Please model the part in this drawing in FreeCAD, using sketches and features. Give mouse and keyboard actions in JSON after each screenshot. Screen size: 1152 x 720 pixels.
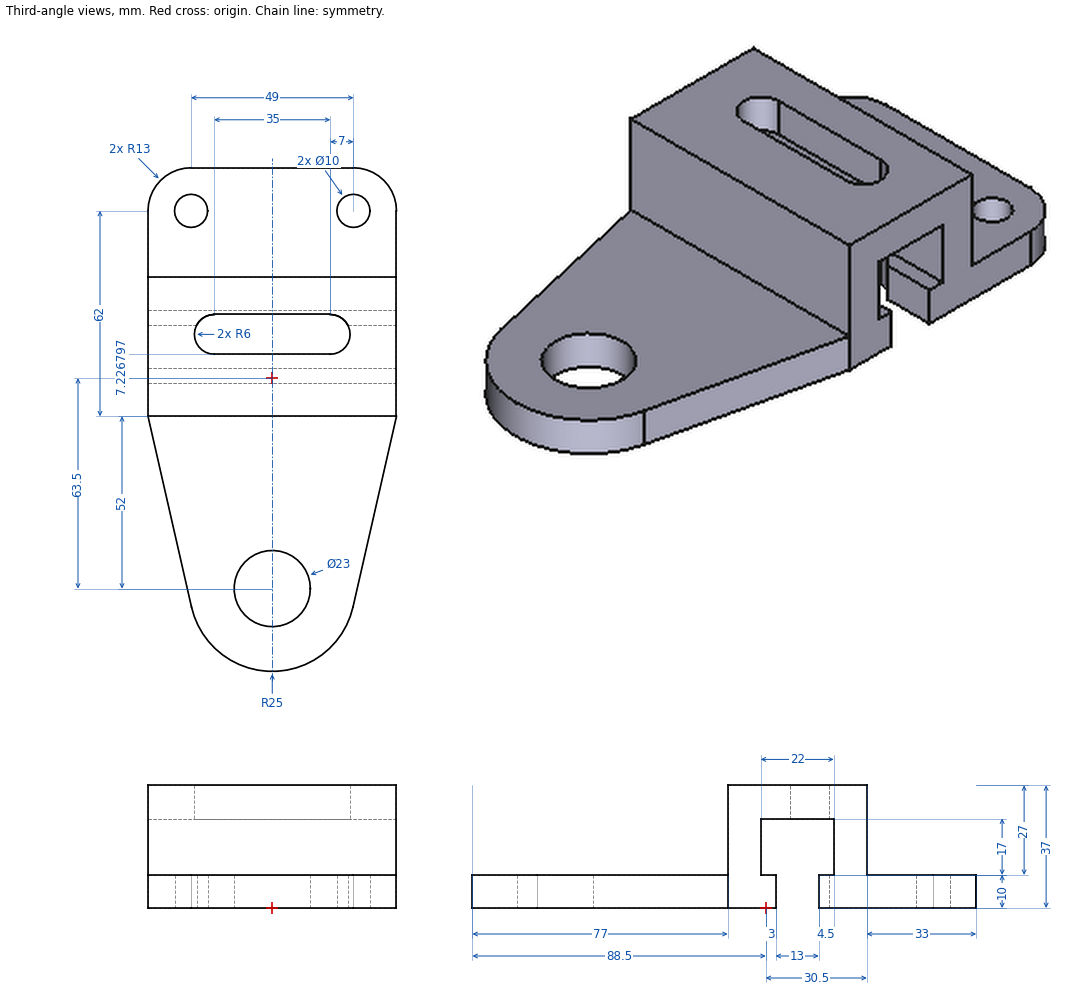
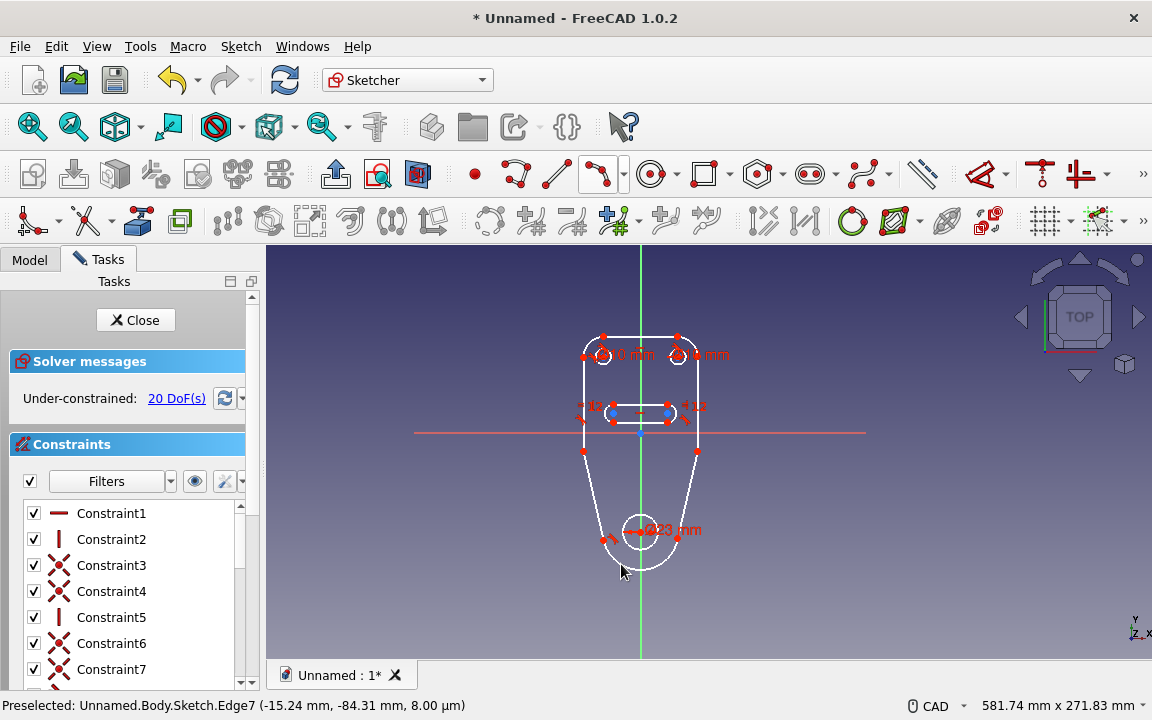
{"action": "left_click", "coordinate": [684, 513]}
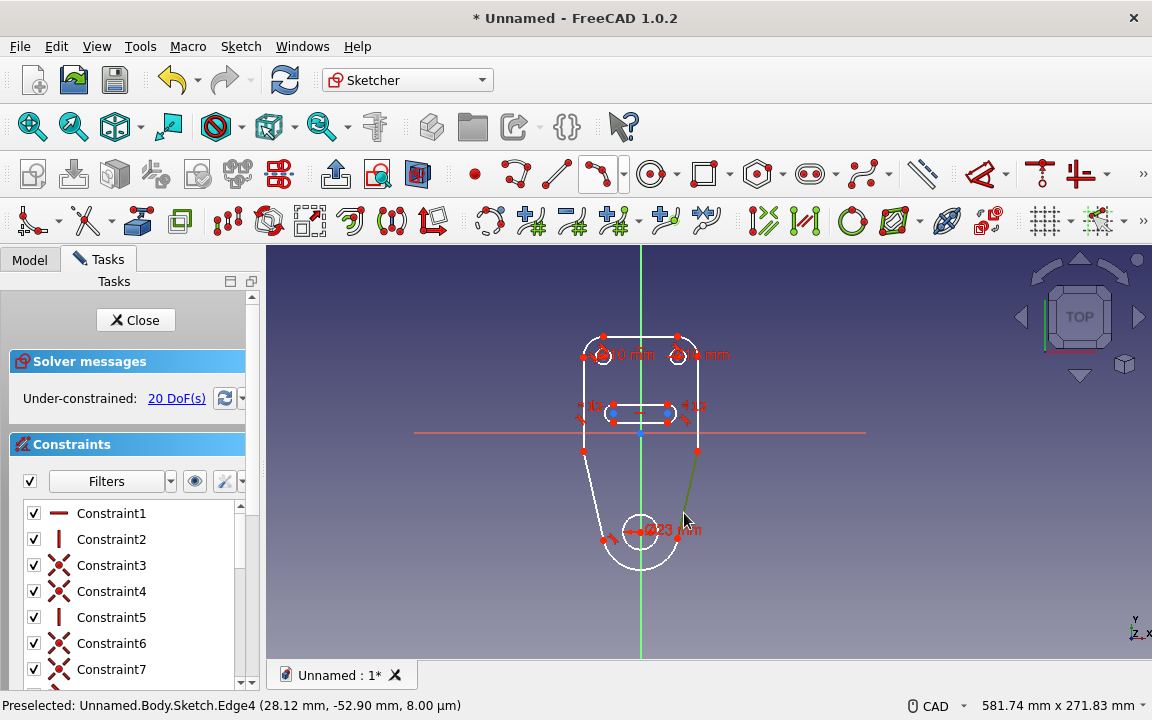
{"action": "left_click", "coordinate": [622, 565]}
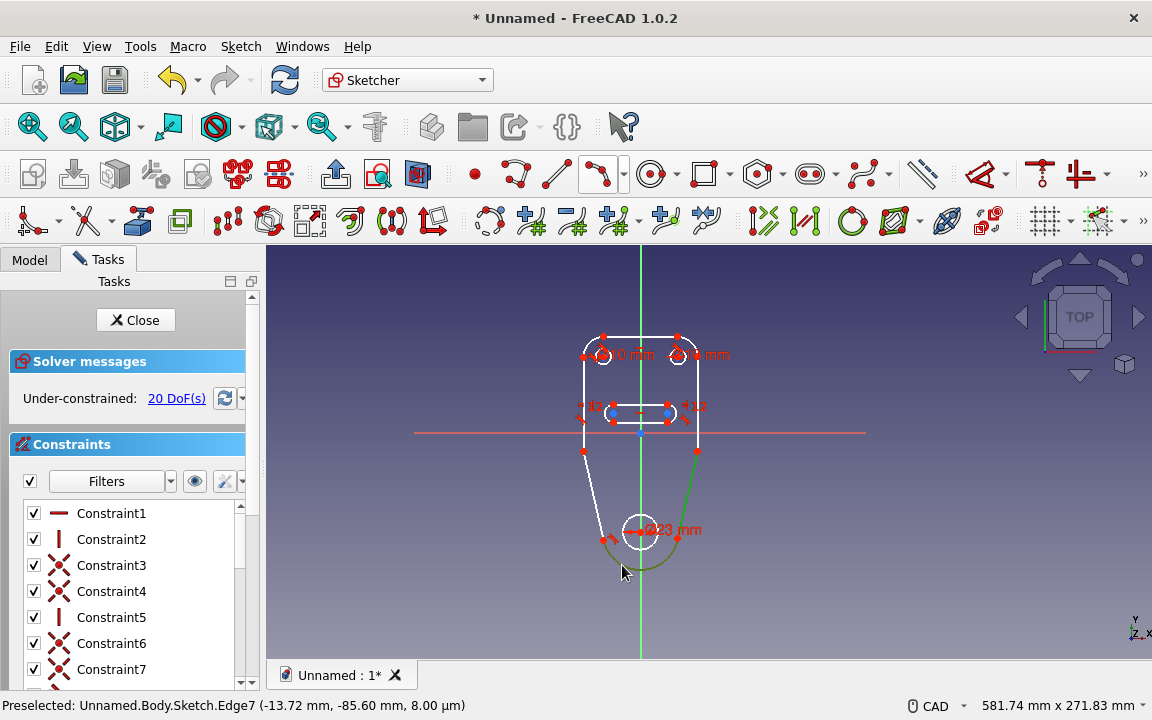
{"action": "key", "text": "t"}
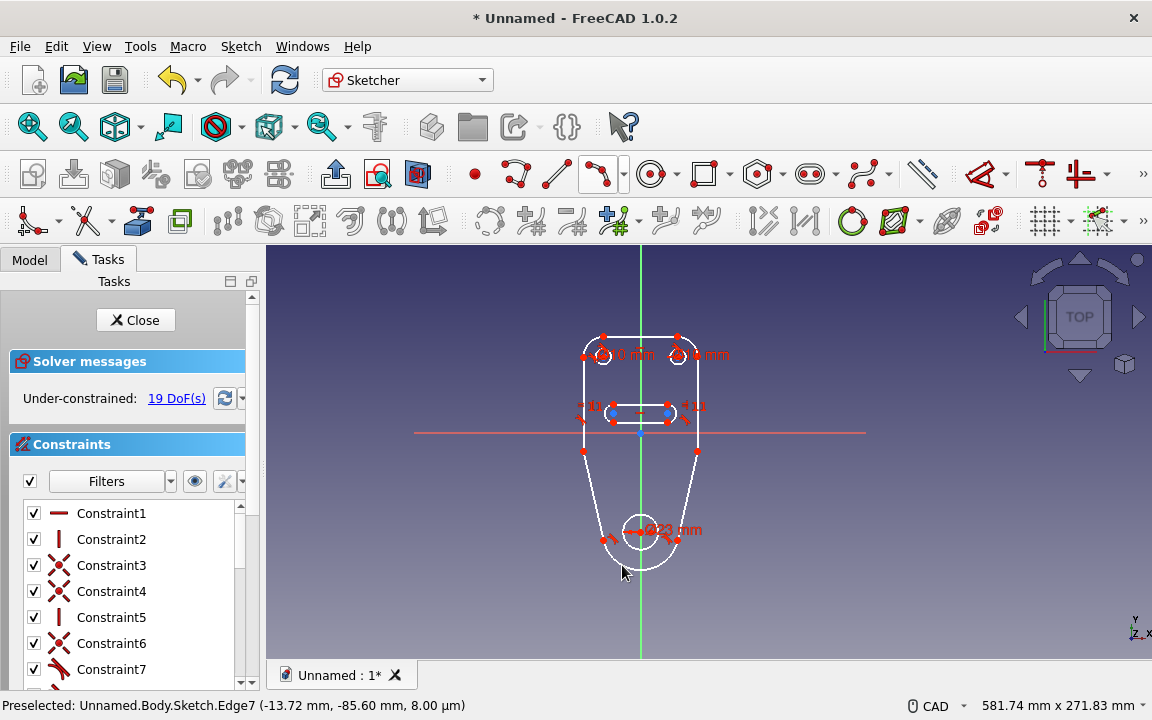
{"action": "scroll", "coordinate": [698, 423], "scroll_direction": "up", "scroll_amount": 2}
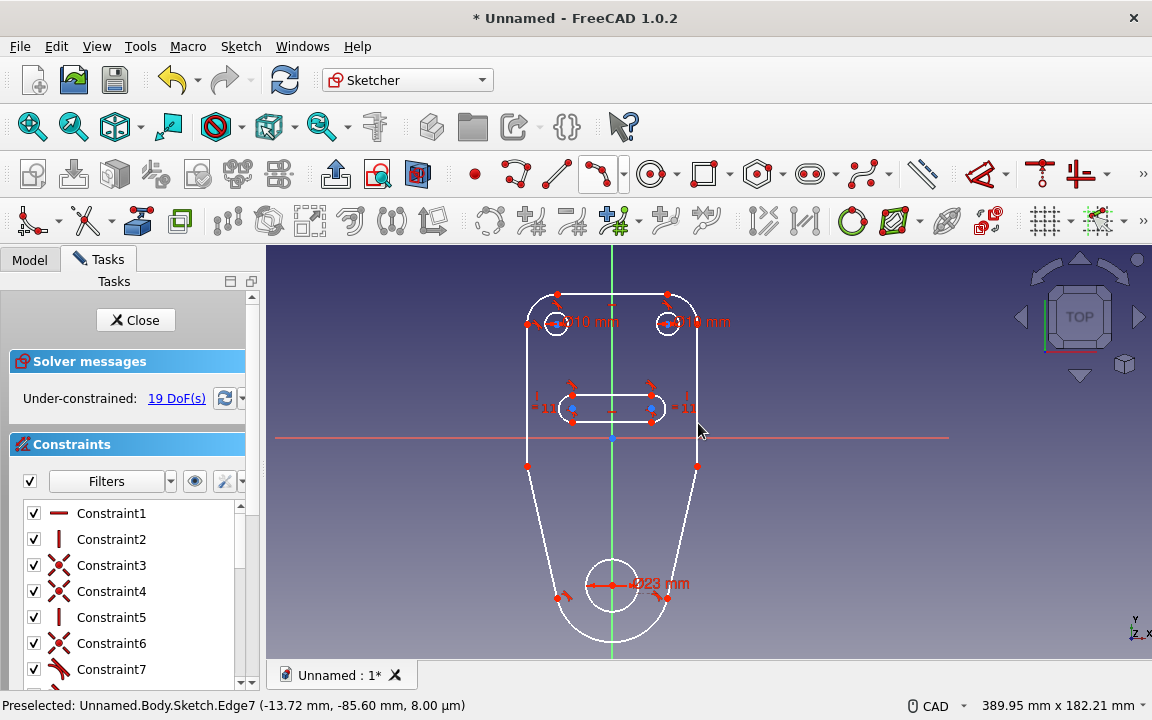
{"action": "left_click", "coordinate": [697, 424]}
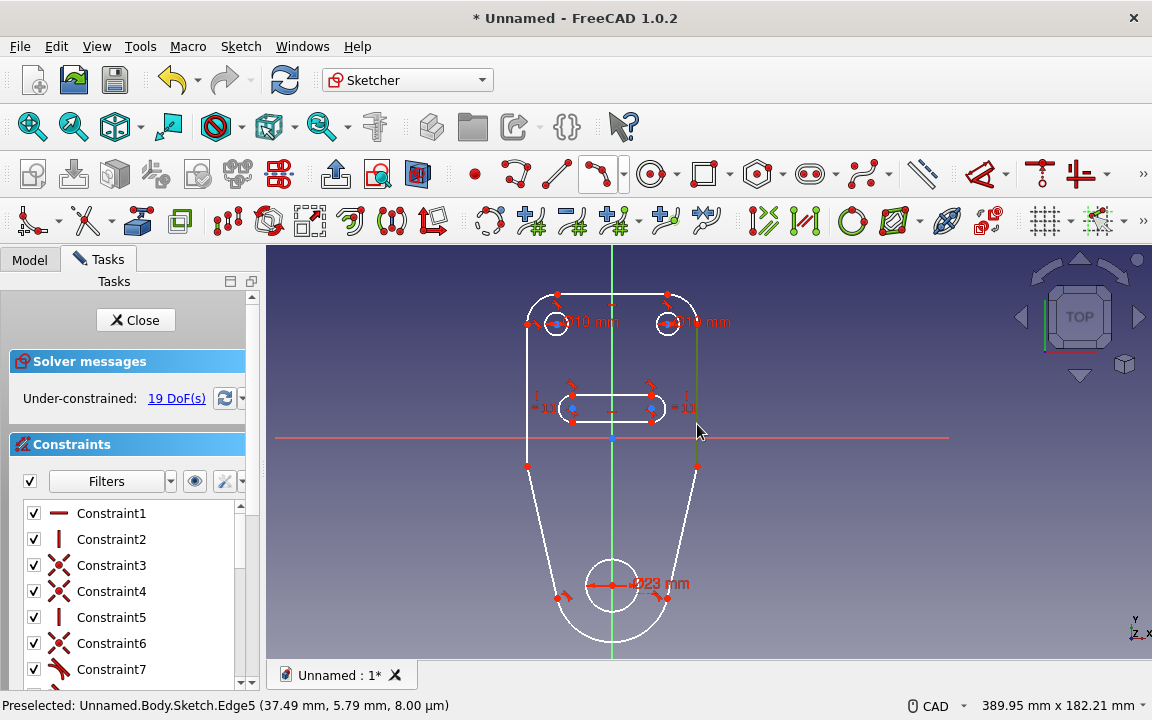
{"action": "left_click", "coordinate": [694, 311]}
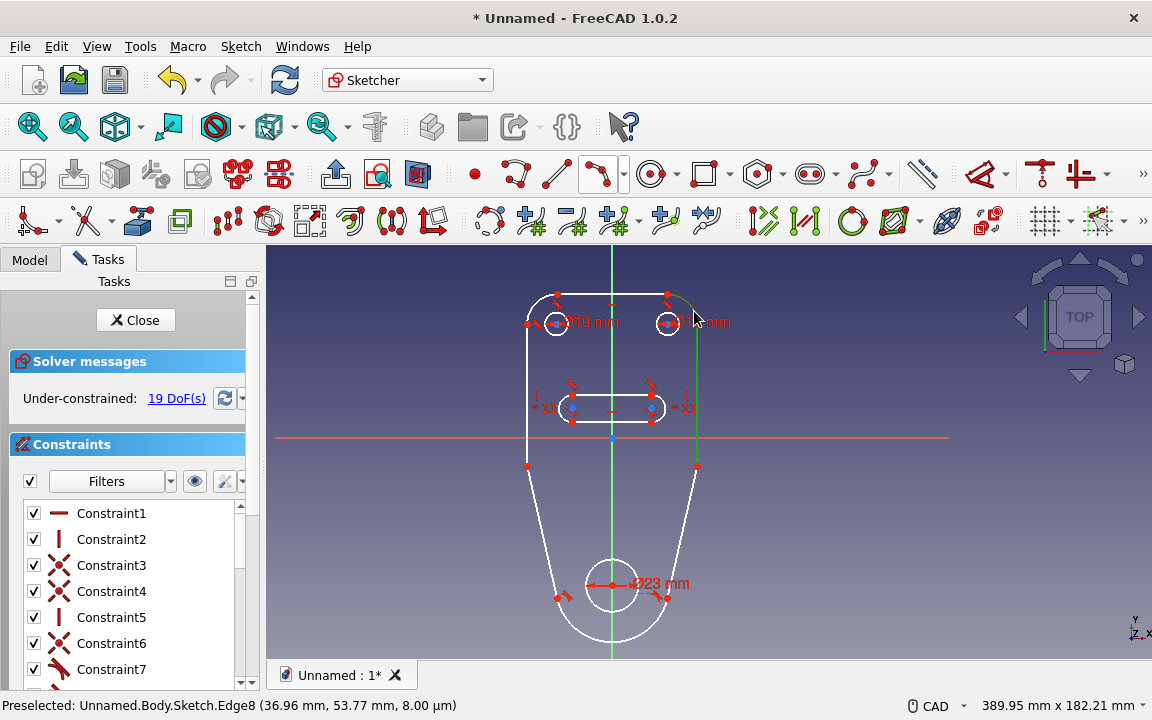
{"action": "key", "text": "t"}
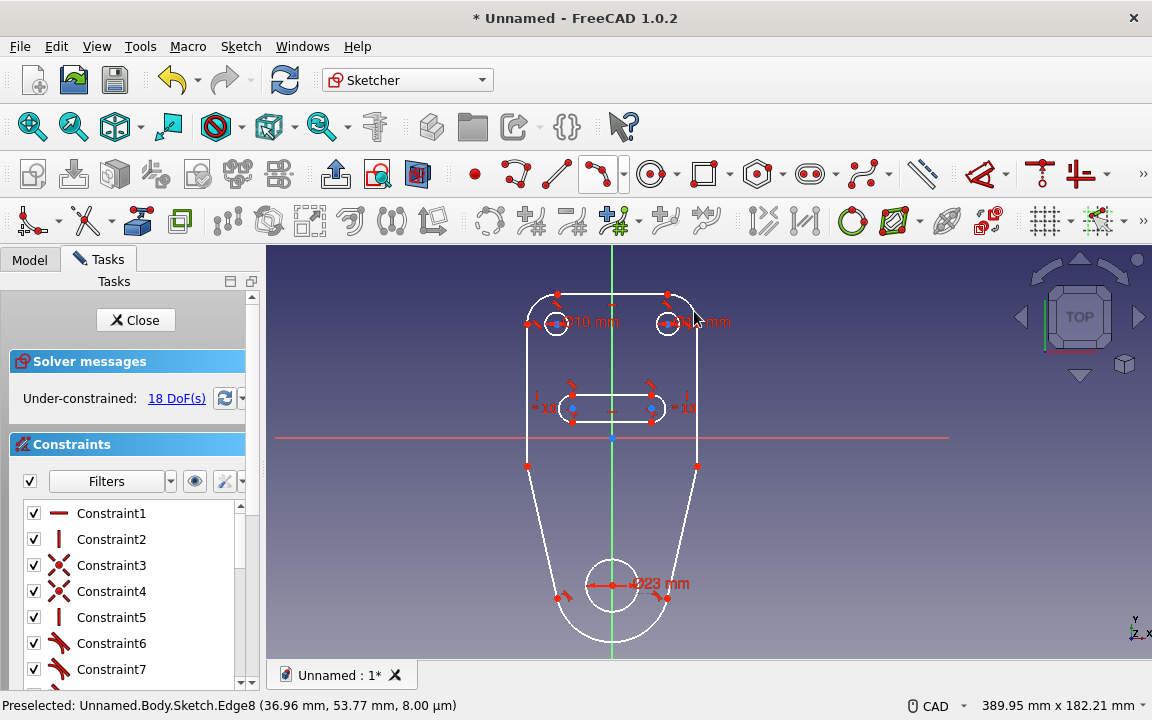
{"action": "left_click", "coordinate": [565, 316]}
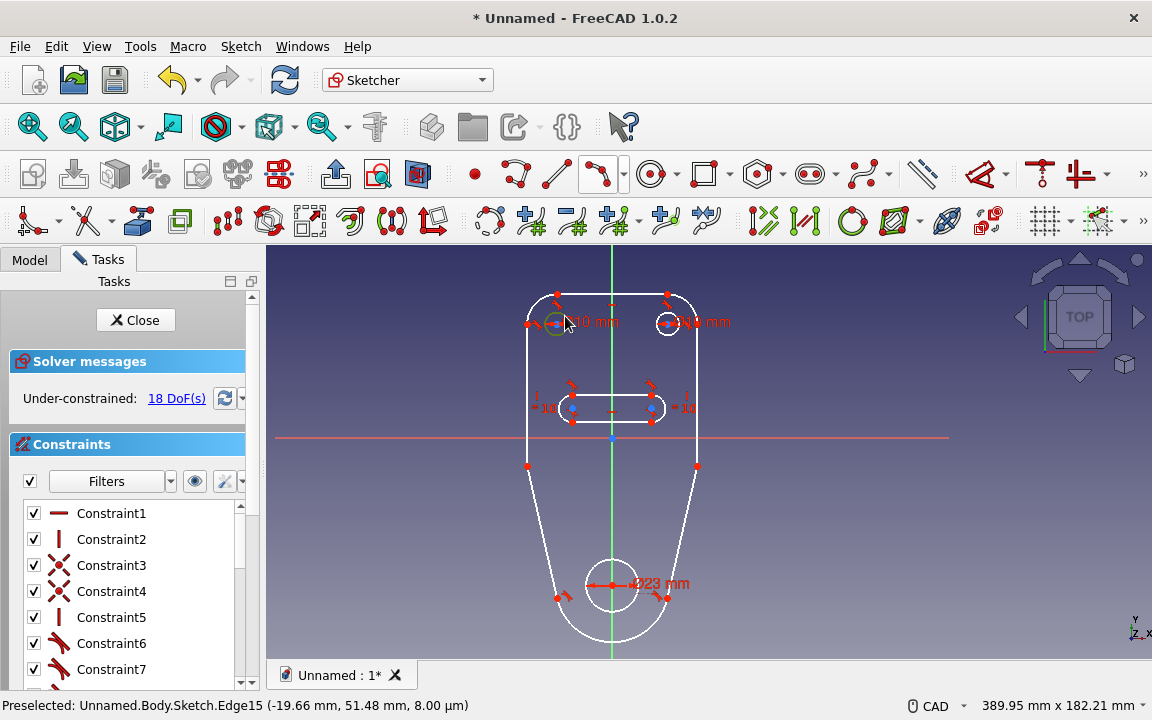
{"action": "left_click", "coordinate": [543, 298]}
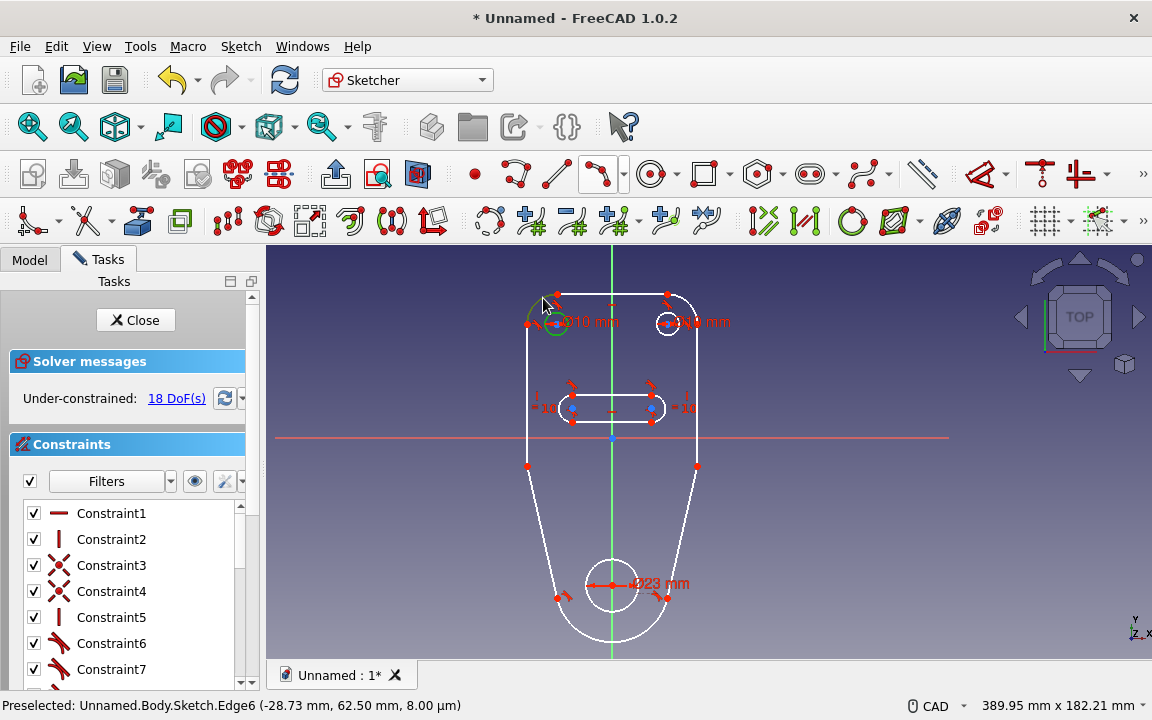
{"action": "left_click", "coordinate": [1040, 174]}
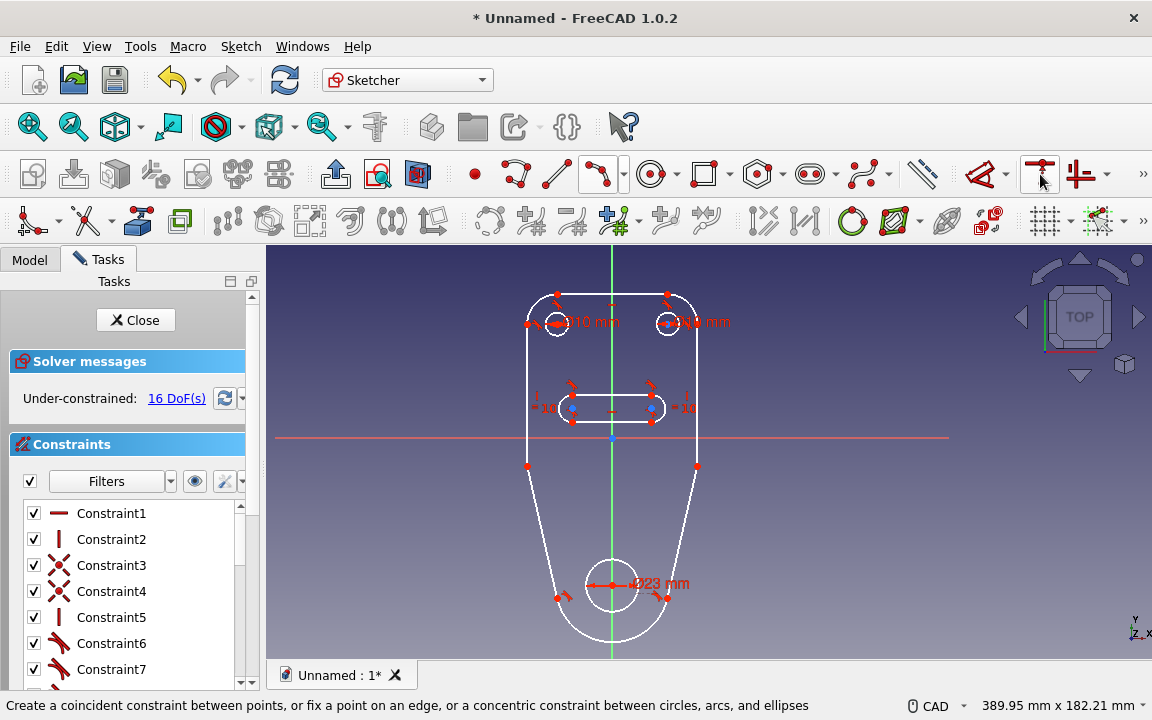
{"action": "left_click", "coordinate": [676, 316]}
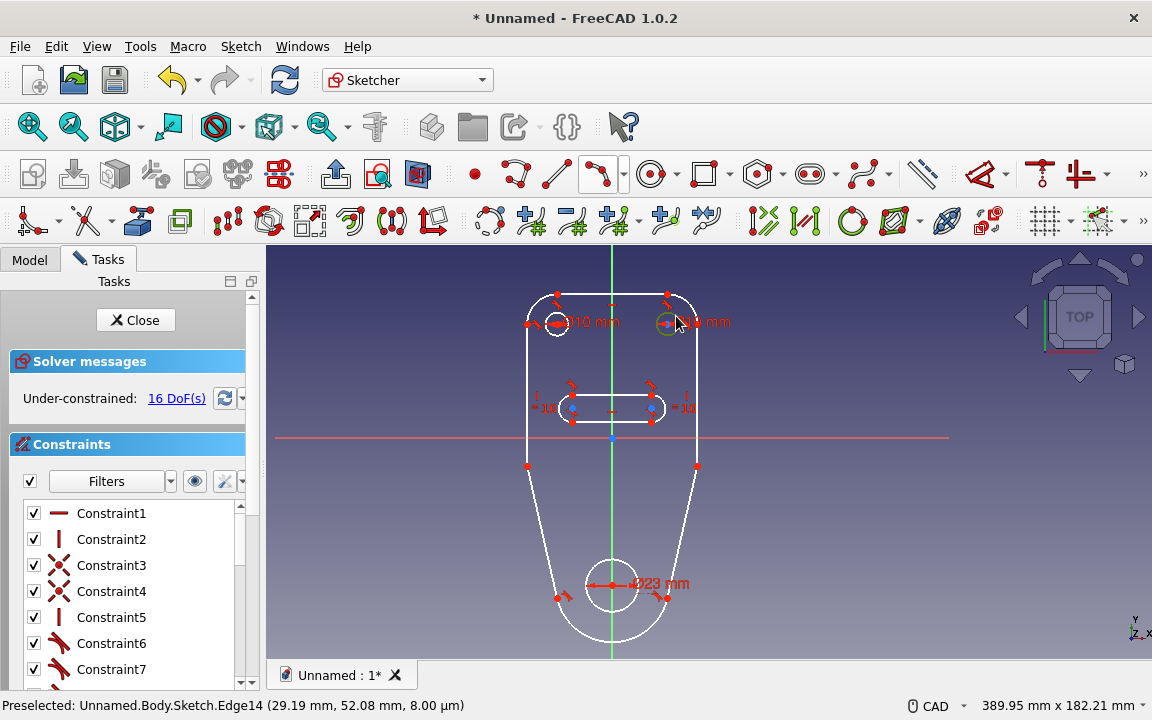
{"action": "left_click", "coordinate": [694, 311]}